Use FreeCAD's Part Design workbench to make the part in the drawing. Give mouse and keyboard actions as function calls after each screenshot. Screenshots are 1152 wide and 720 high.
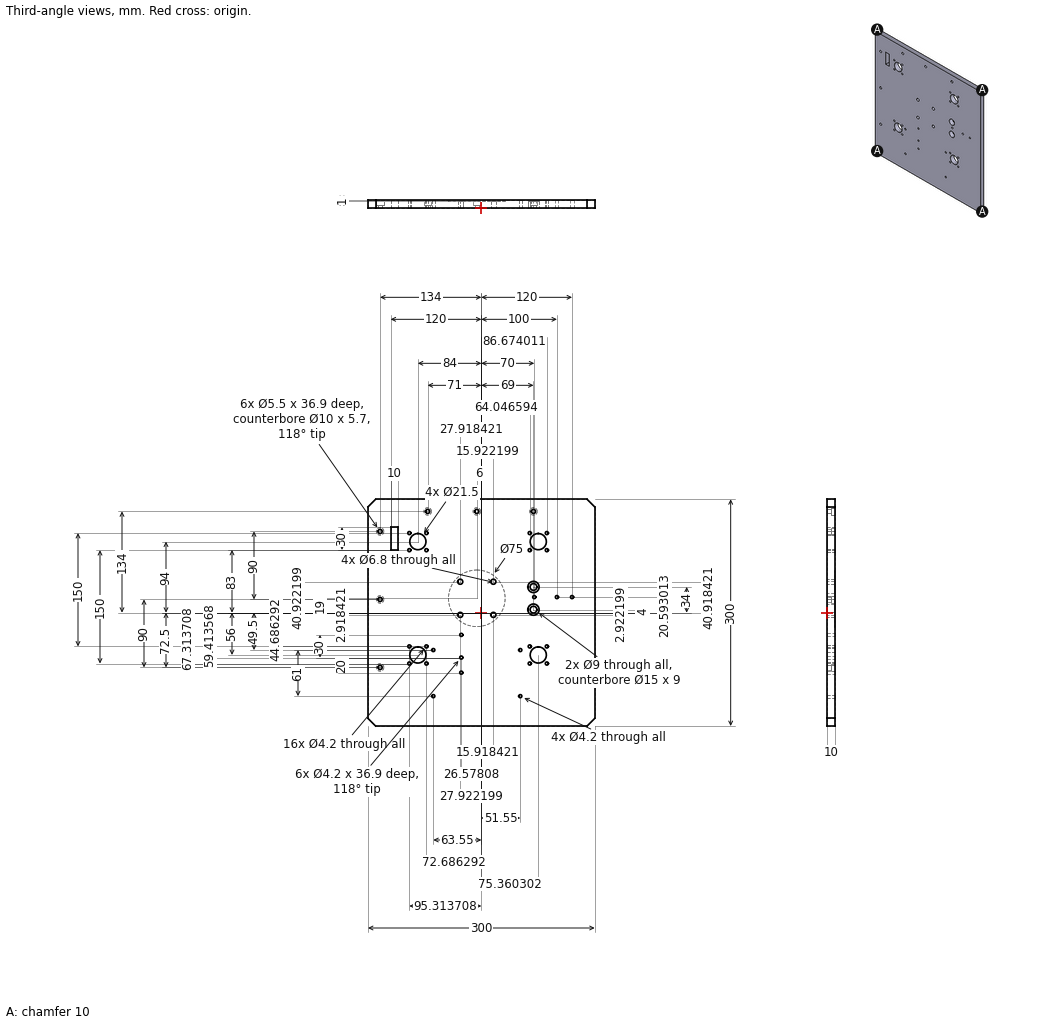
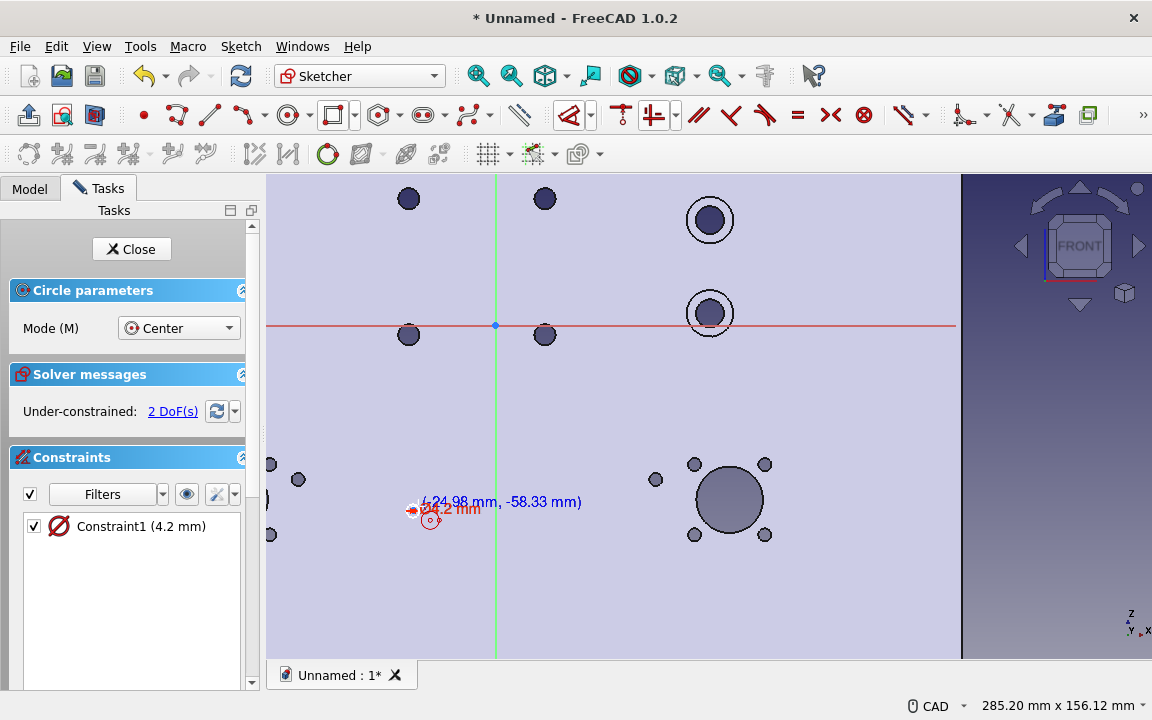
scroll(806, 262, up, 7)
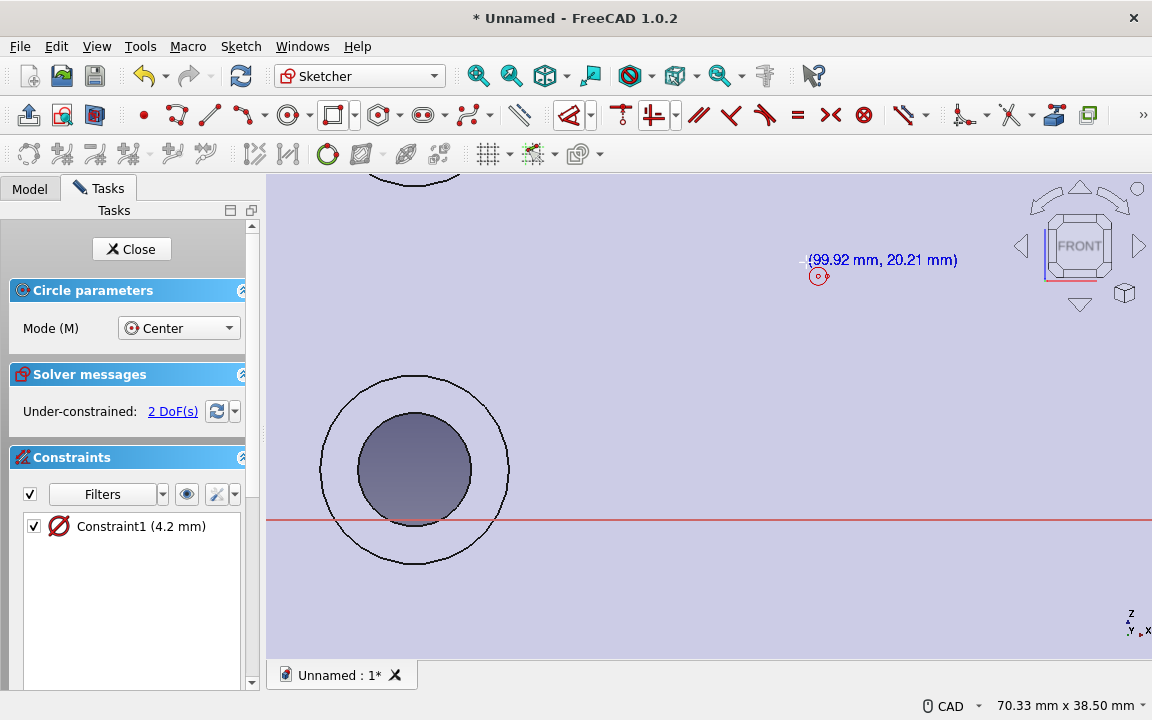
scroll(806, 261, down, 7)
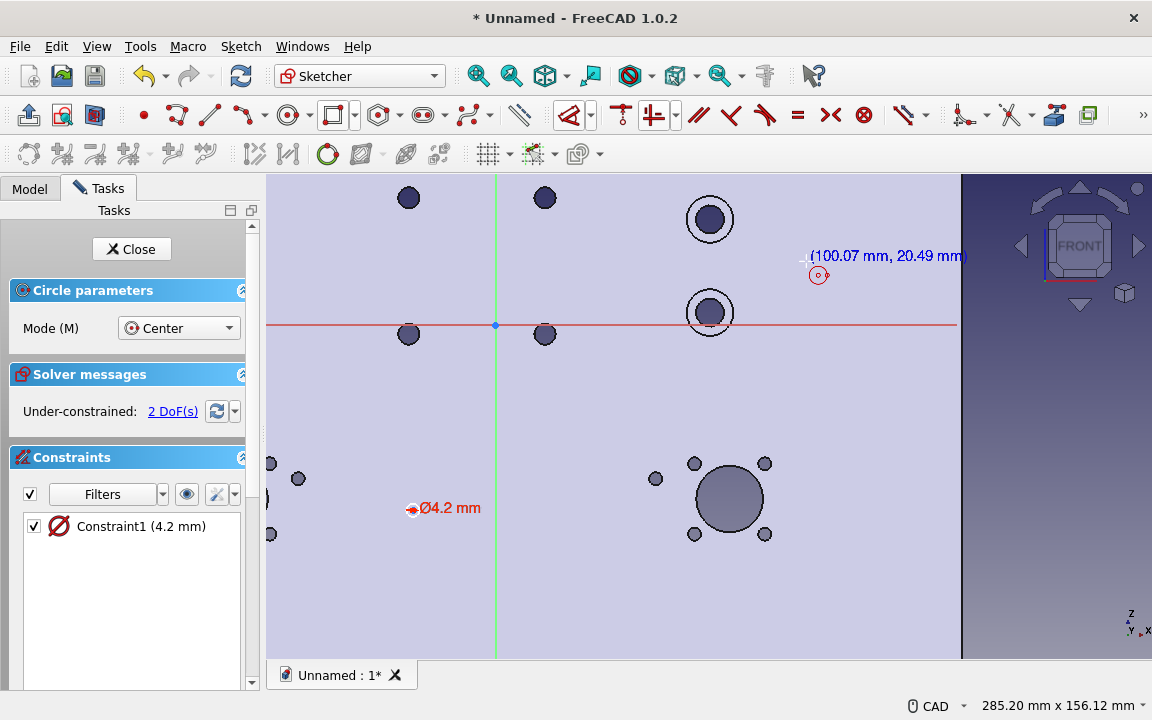
click(806, 261)
move(811, 256)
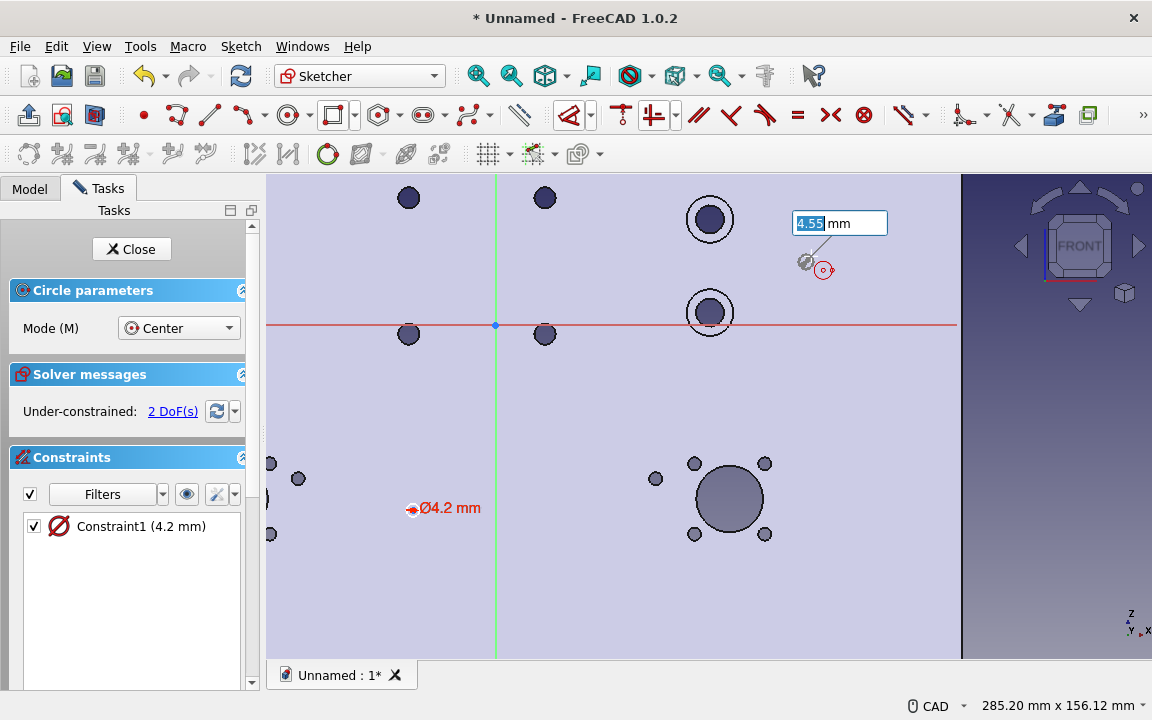
text(4.2)
key(Return)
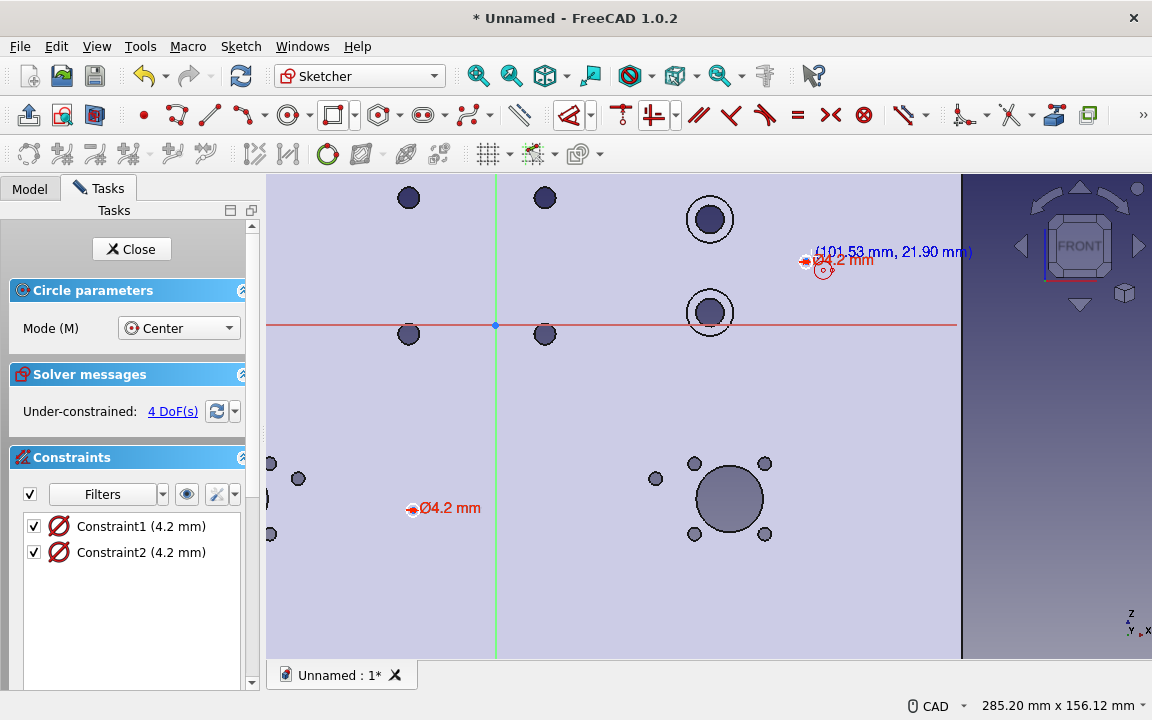
scroll(413, 572, up, 7)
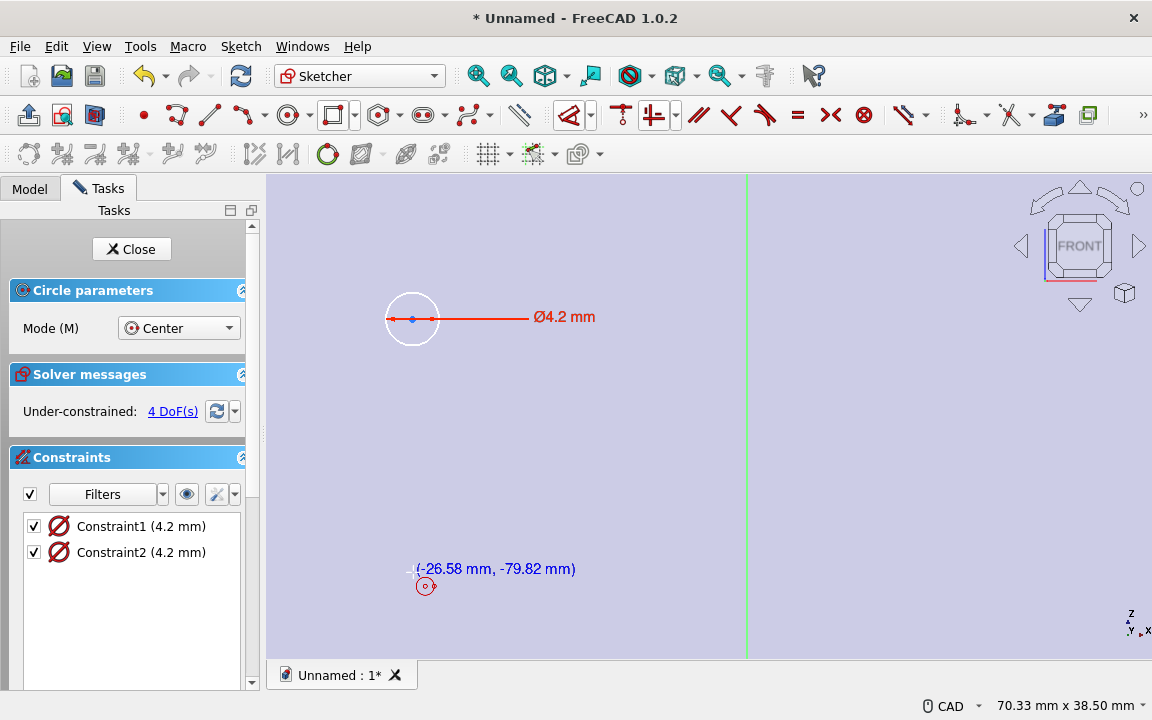
scroll(413, 573, down, 7)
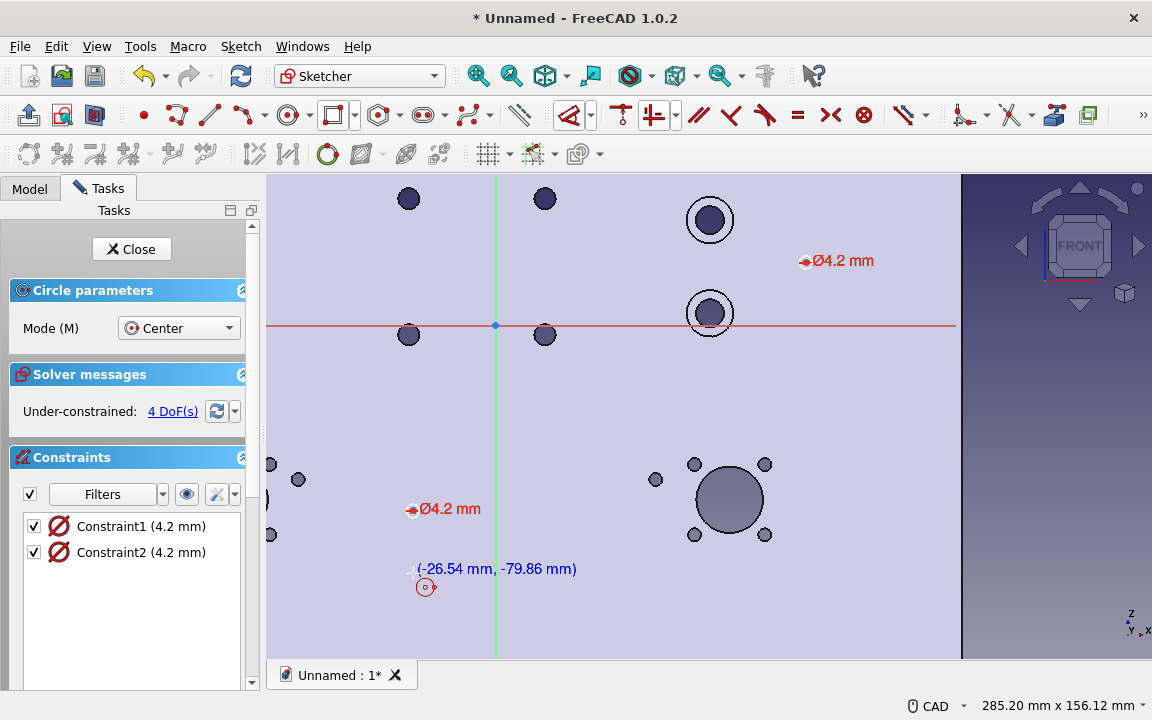
click(413, 572)
move(418, 568)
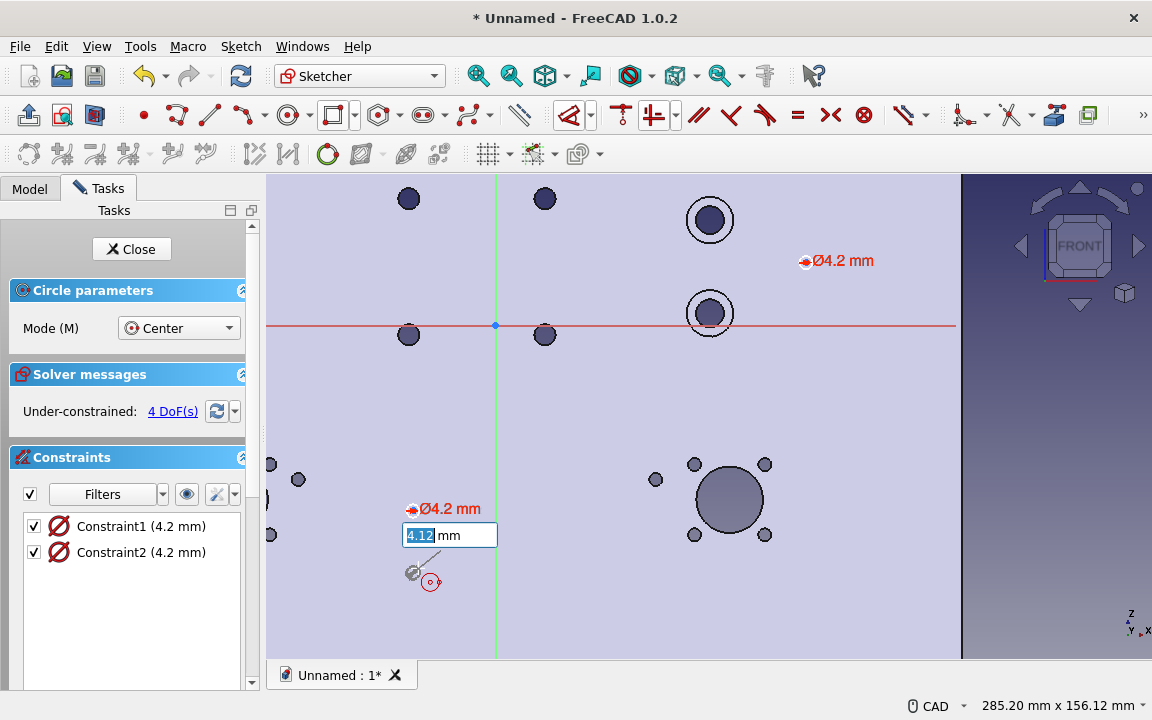
text(4.2)
key(Return)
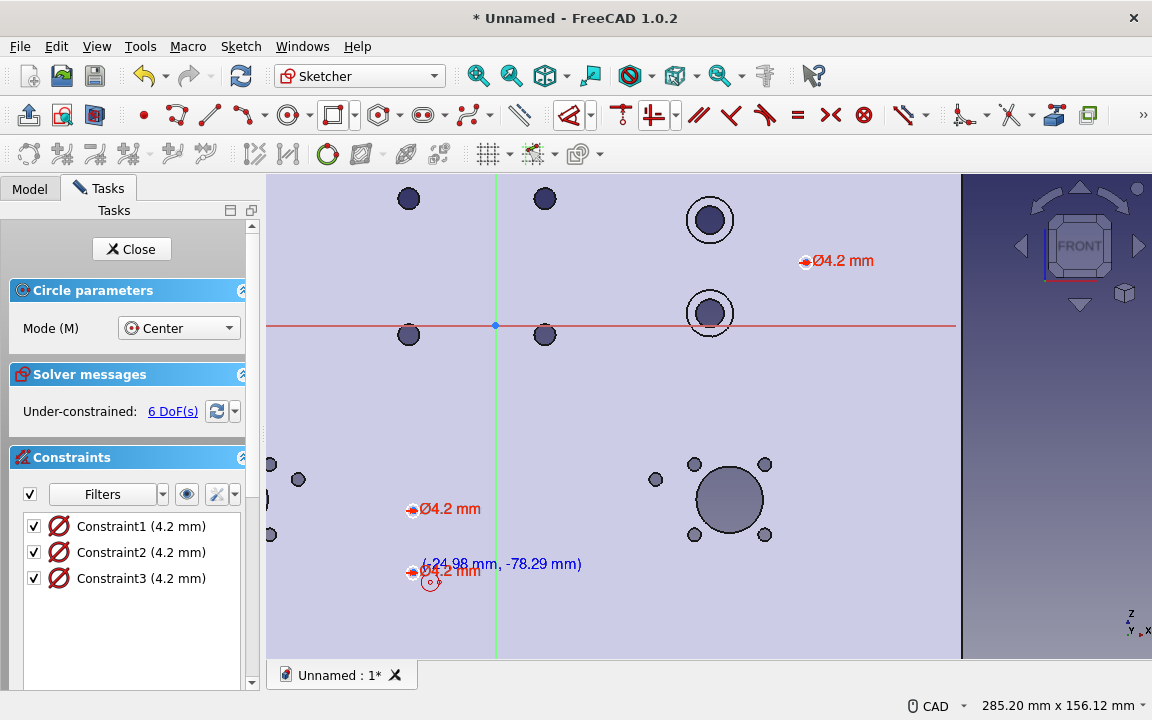
scroll(413, 417, up, 7)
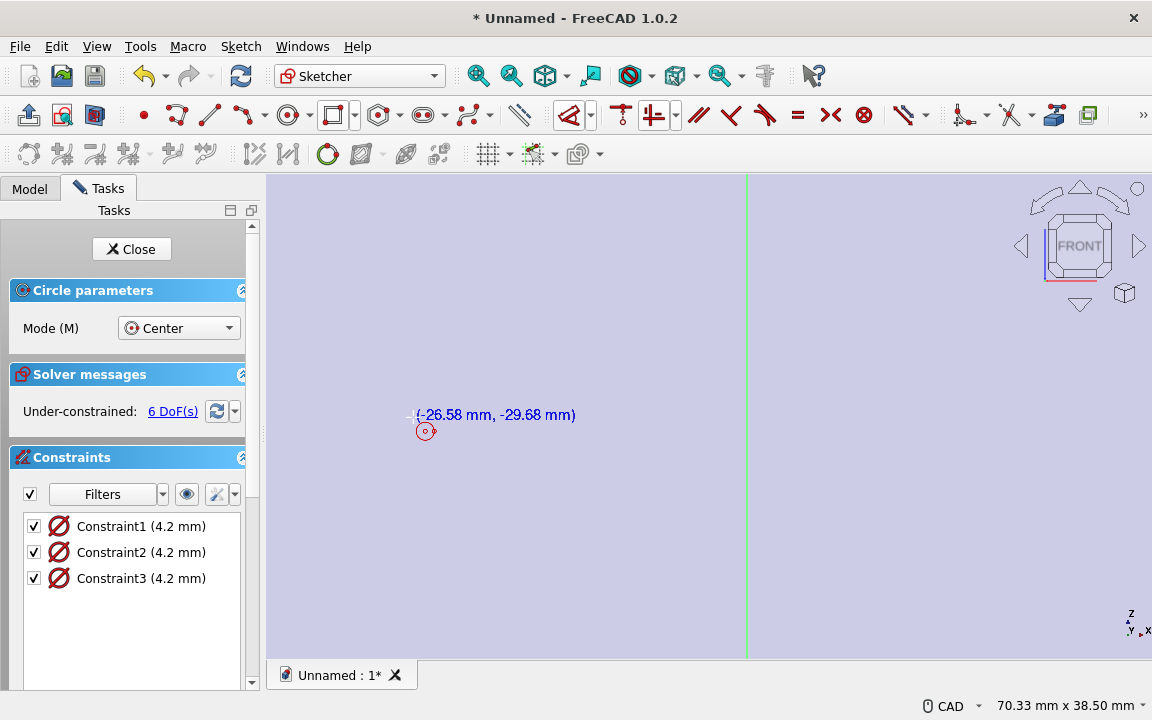
scroll(413, 417, down, 7)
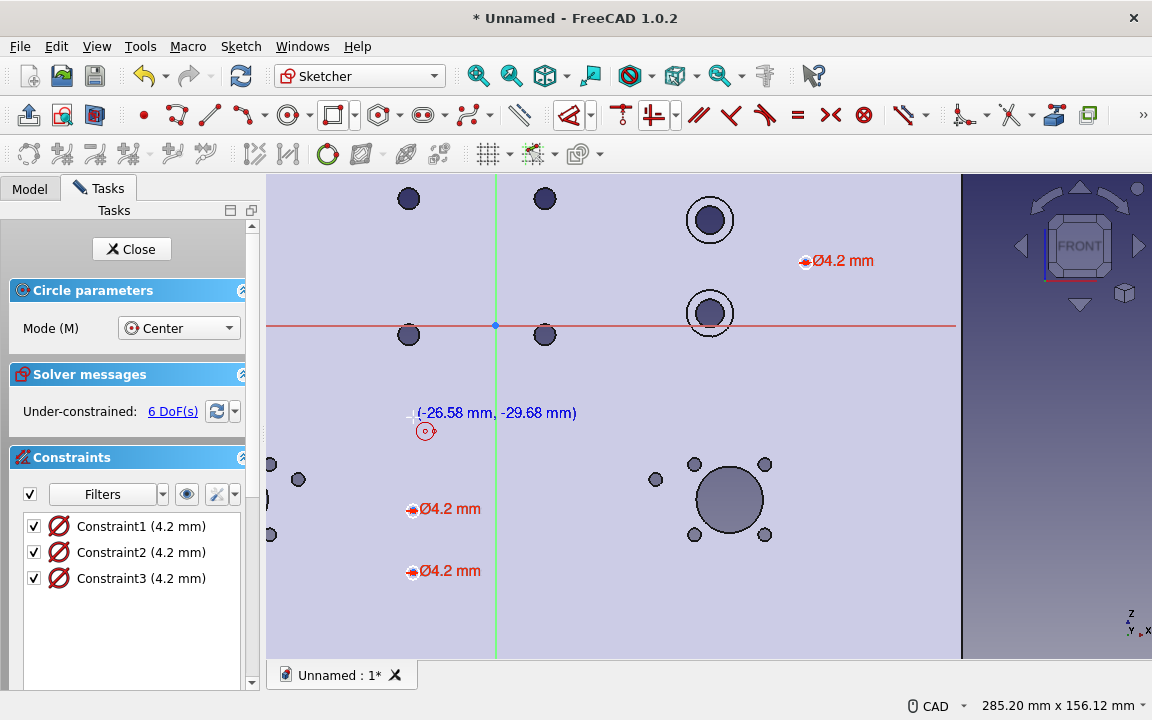
click(413, 417)
move(418, 413)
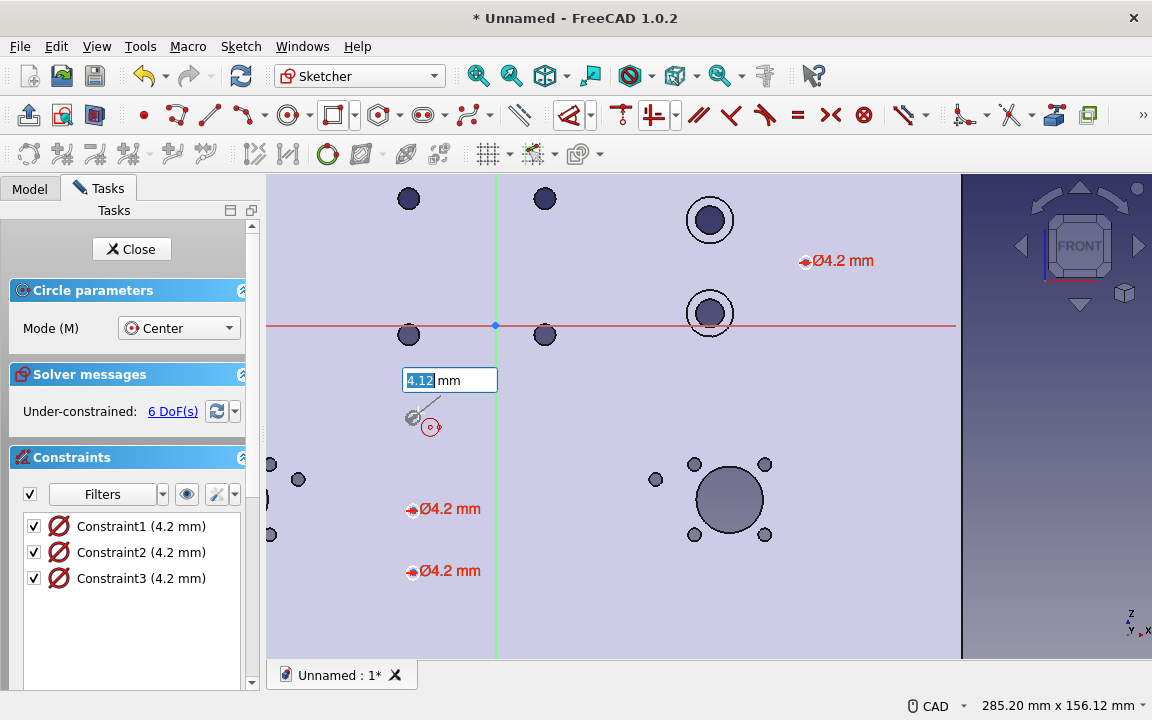
text(4.2)
key(Return)